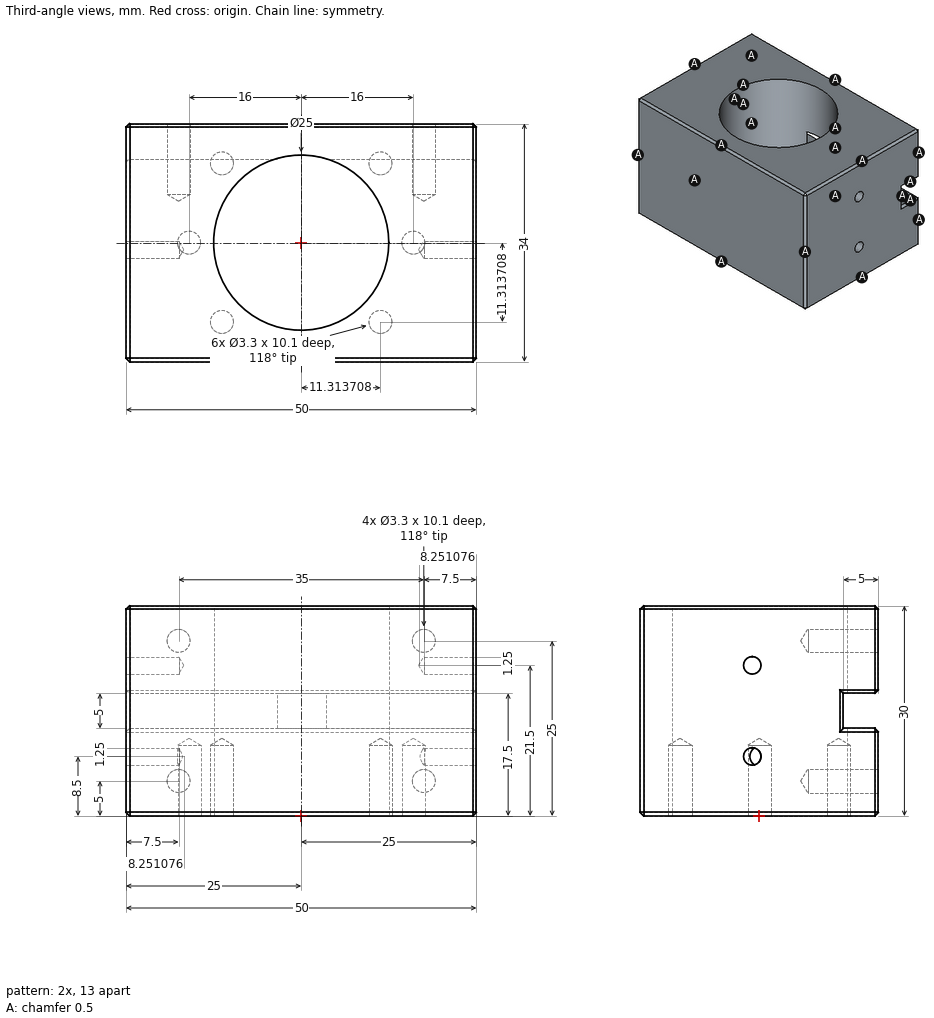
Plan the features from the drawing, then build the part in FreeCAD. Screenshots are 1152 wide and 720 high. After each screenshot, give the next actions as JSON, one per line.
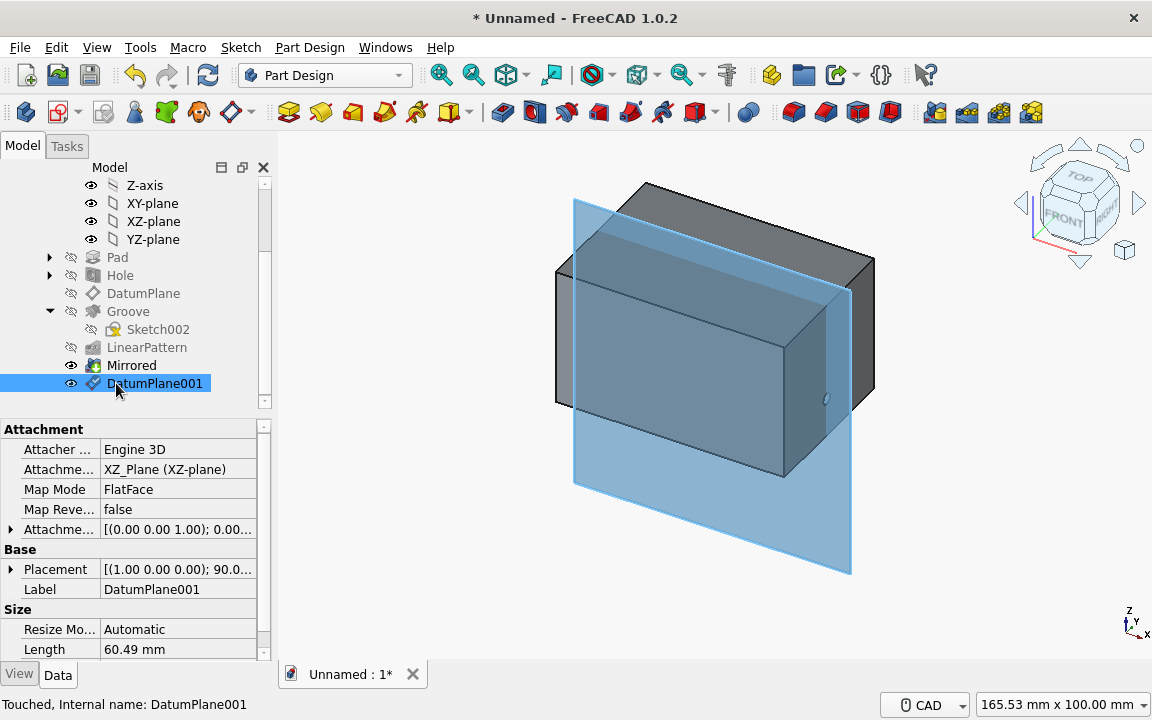
{"action": "left_click", "coordinate": [58, 112]}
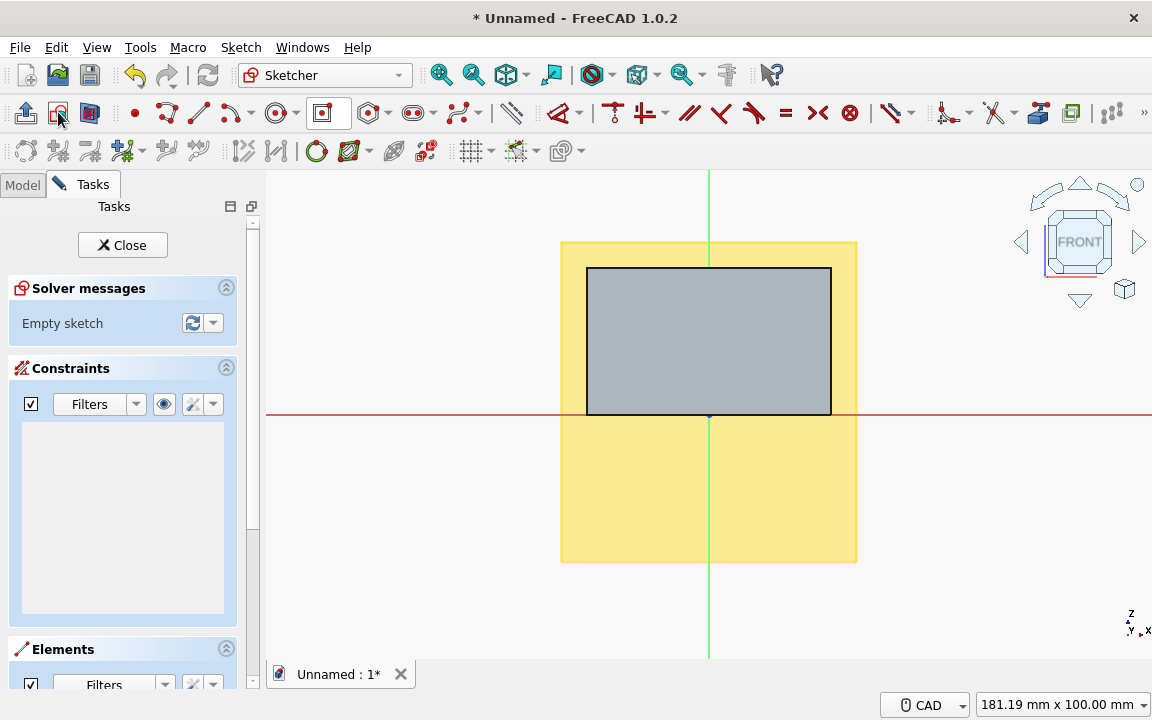
{"action": "key", "text": "q s"}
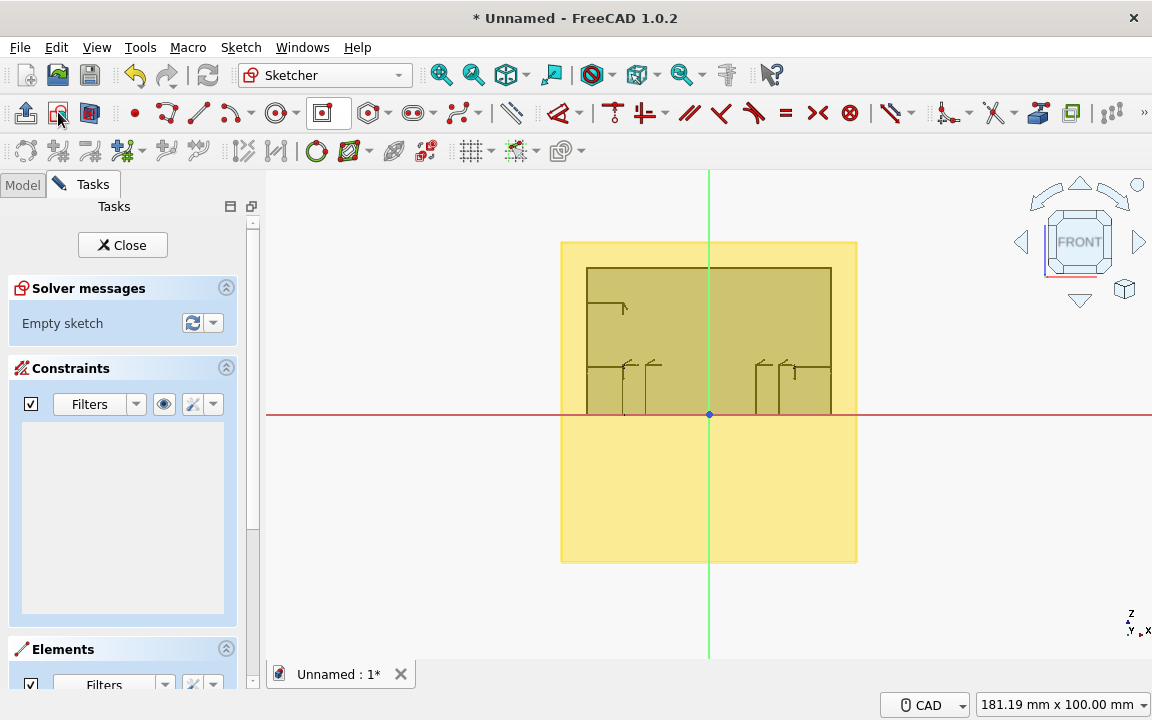
{"action": "scroll", "coordinate": [858, 327], "scroll_direction": "up", "scroll_amount": 5}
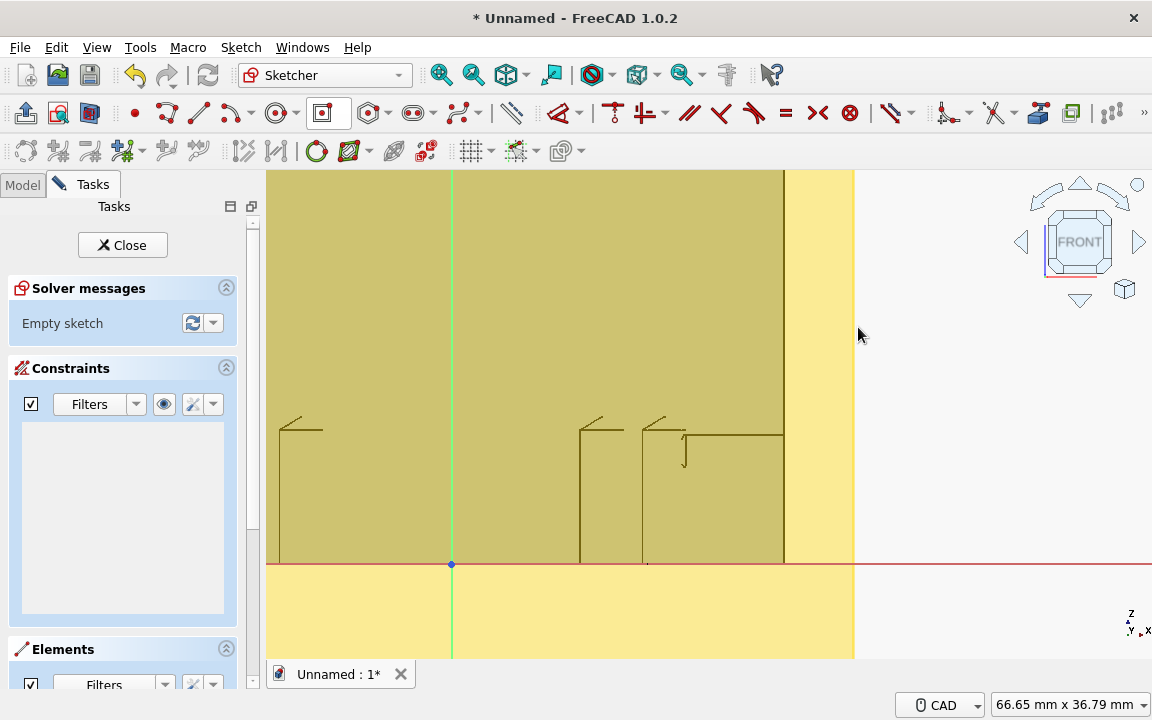
{"action": "left_click", "coordinate": [168, 114]}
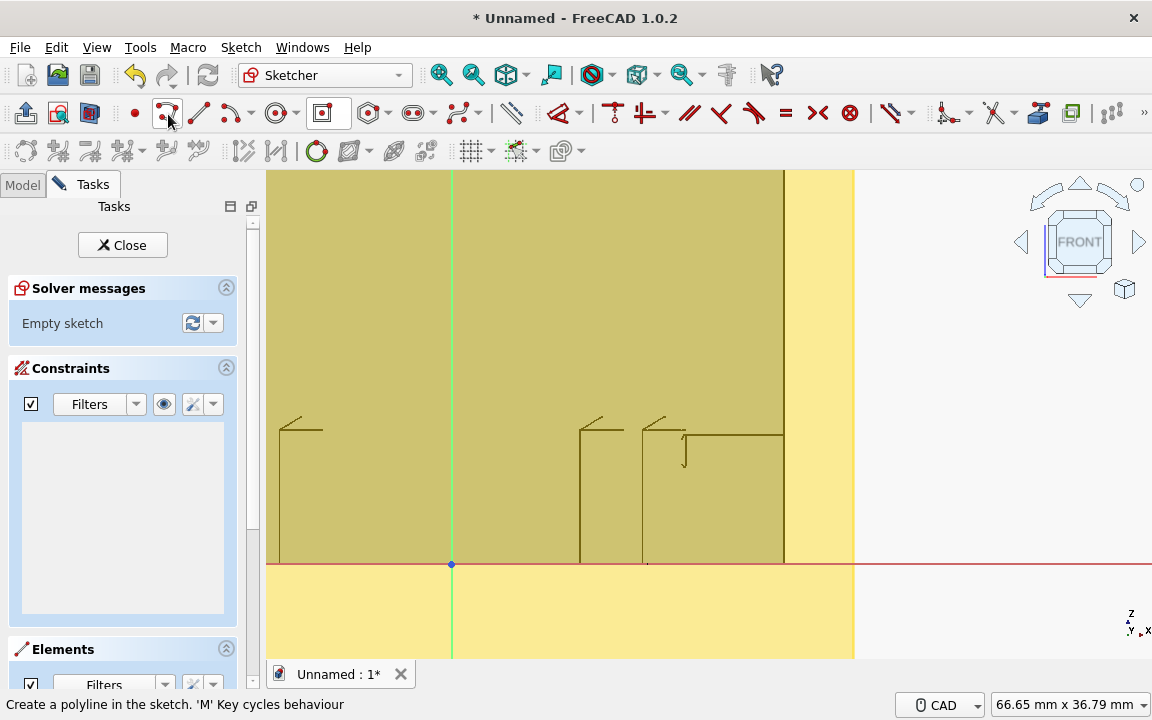
{"action": "left_click", "coordinate": [674, 279]}
{"action": "left_click", "coordinate": [684, 262]}
{"action": "left_click", "coordinate": [784, 262]}
{"action": "left_click", "coordinate": [784, 279]}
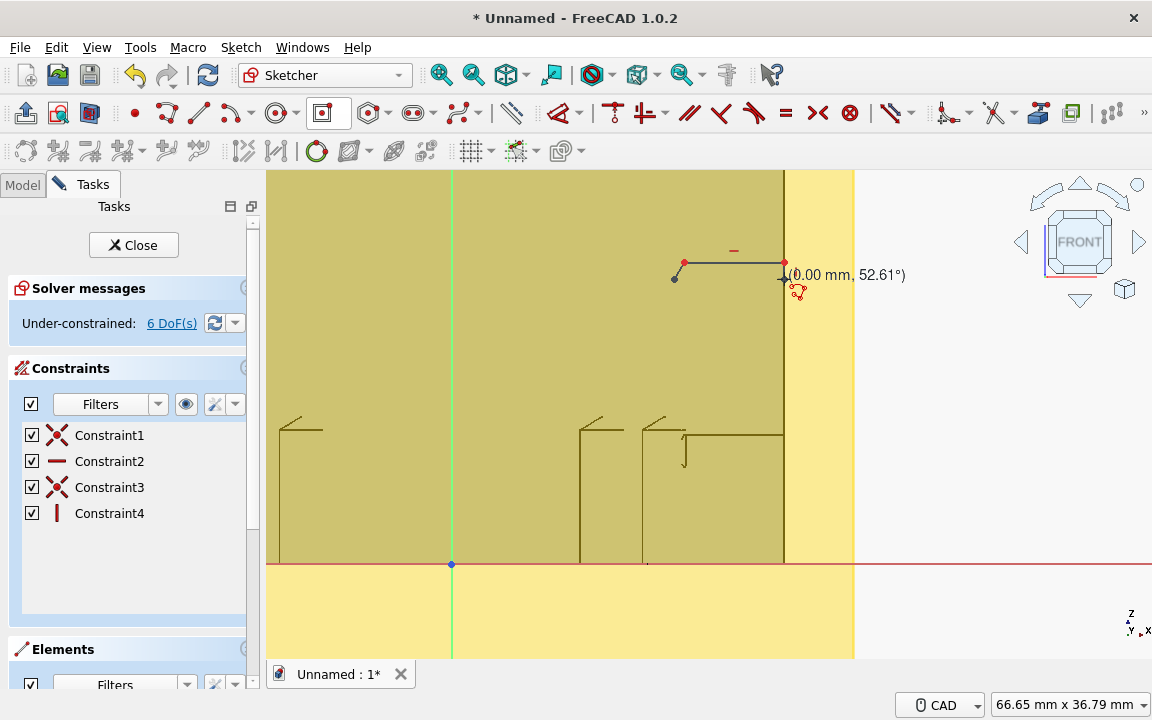
{"action": "scroll", "coordinate": [674, 279], "scroll_direction": "up", "scroll_amount": 3}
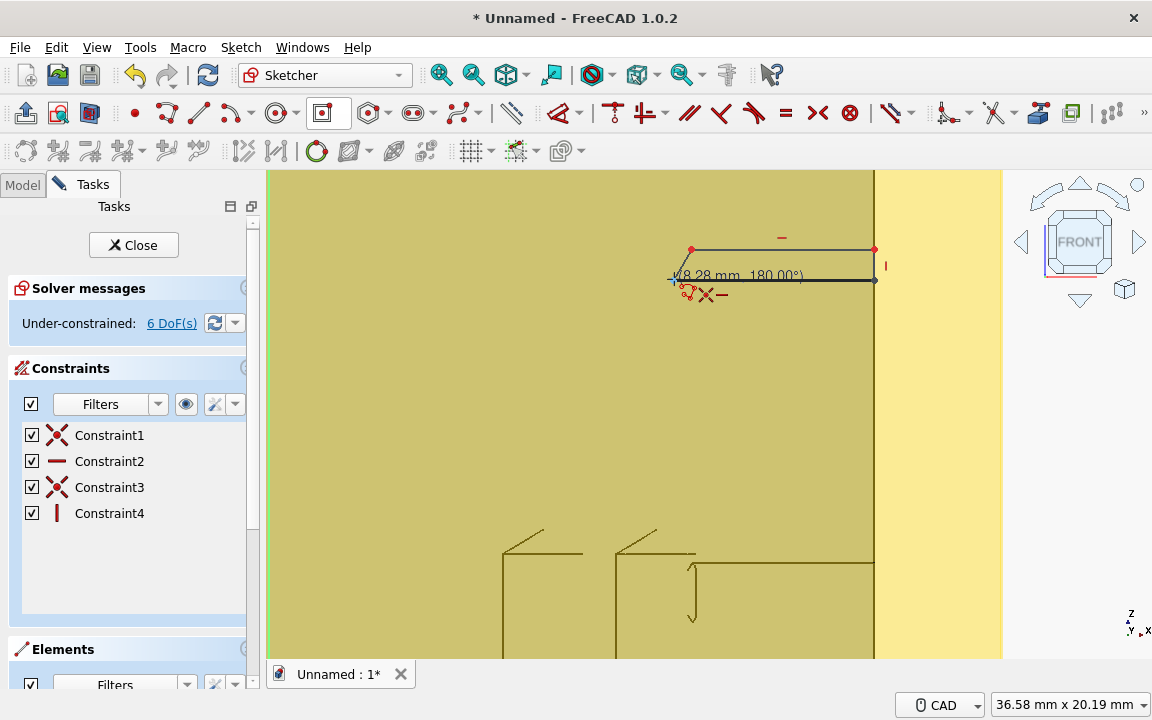
{"action": "left_click", "coordinate": [674, 281]}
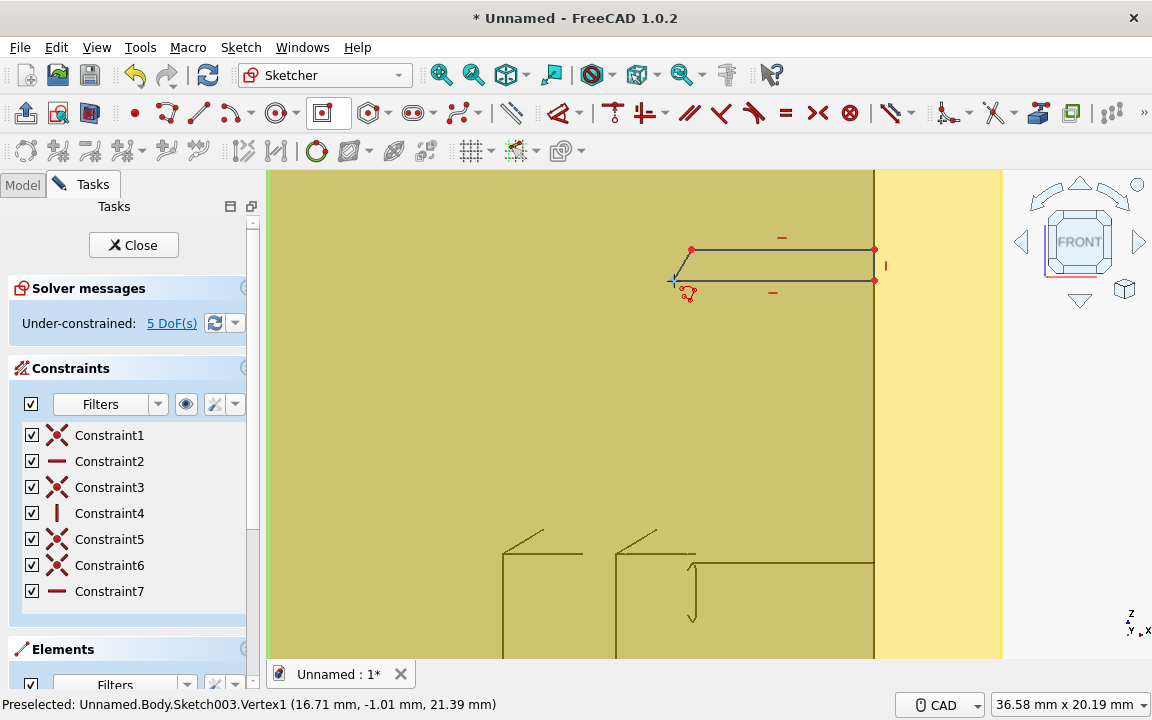
{"action": "key", "text": "g l"}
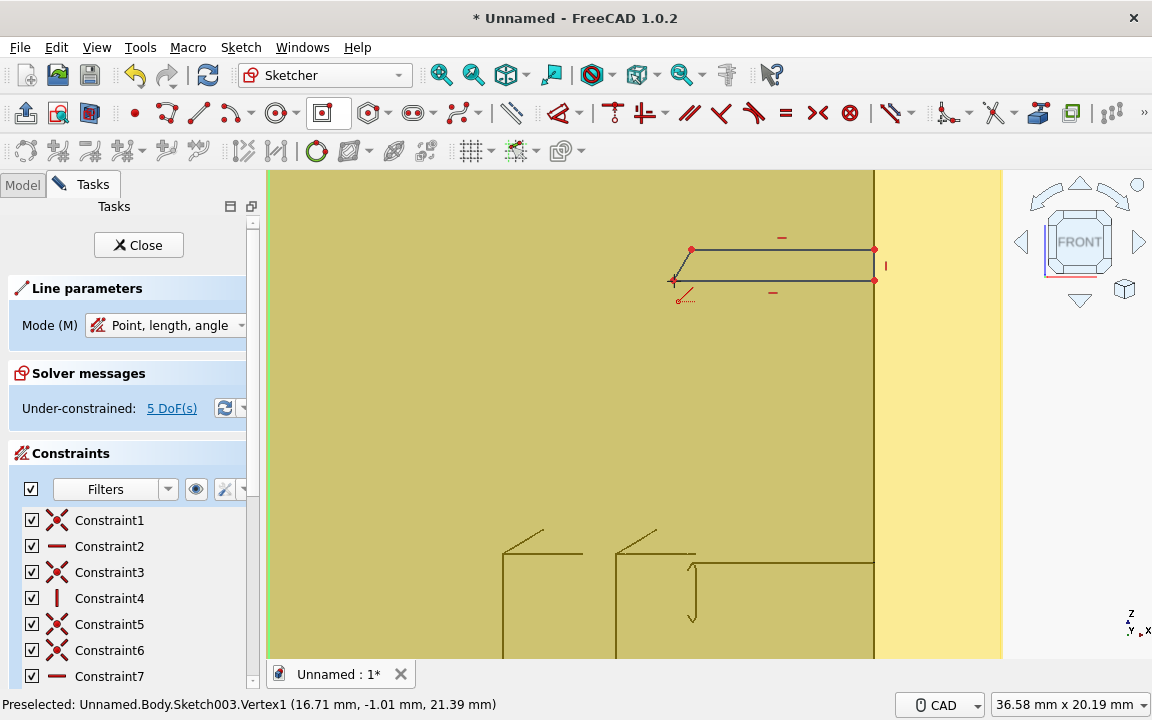
{"action": "left_click", "coordinate": [894, 278]}
{"action": "left_click", "coordinate": [954, 278]}
{"action": "key", "text": "Escape"}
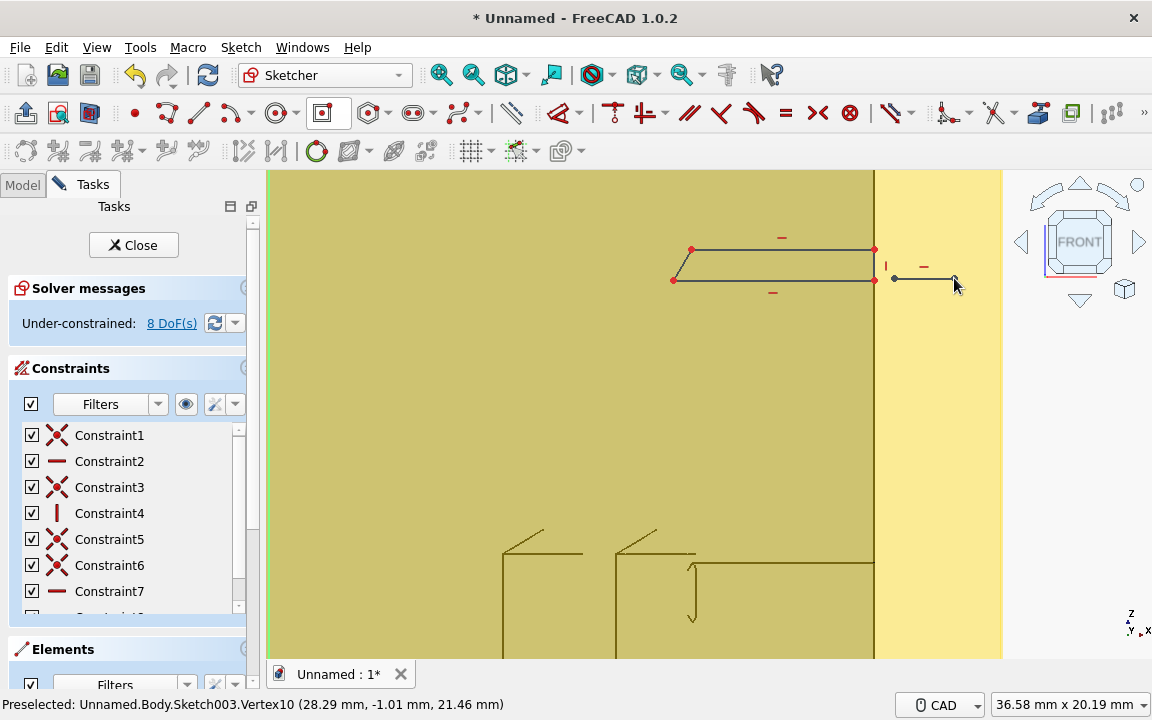
{"action": "left_click", "coordinate": [912, 279]}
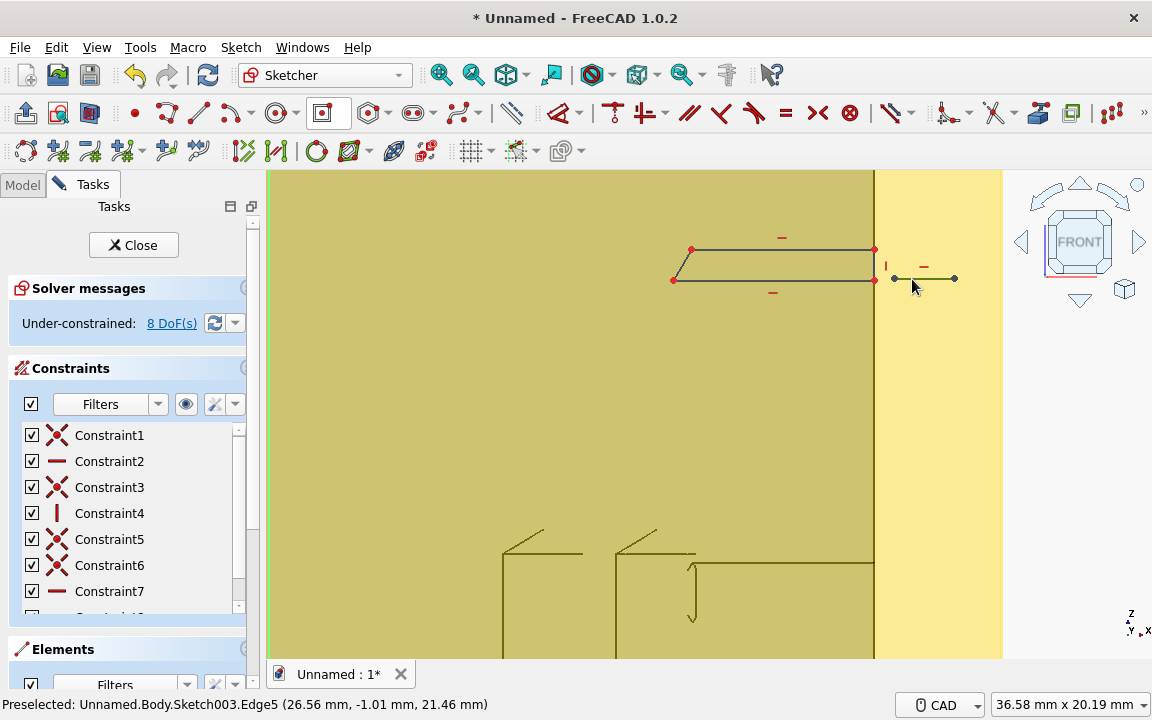
{"action": "left_click", "coordinate": [512, 114]}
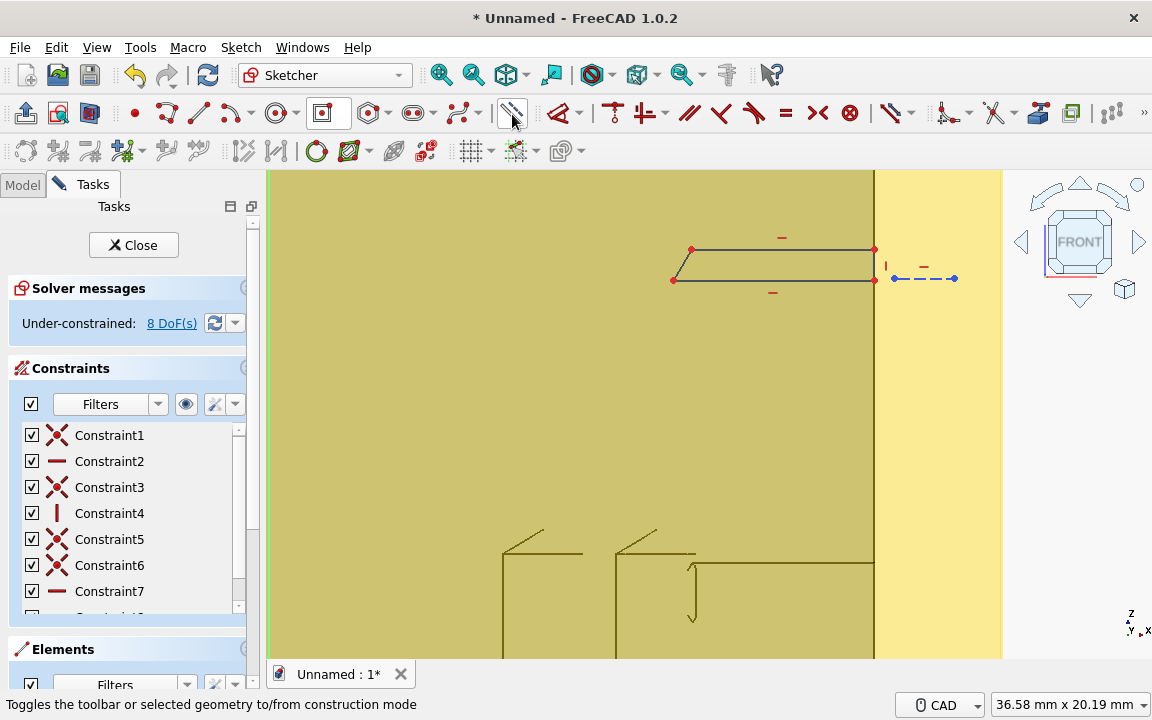
{"action": "key", "text": "d"}